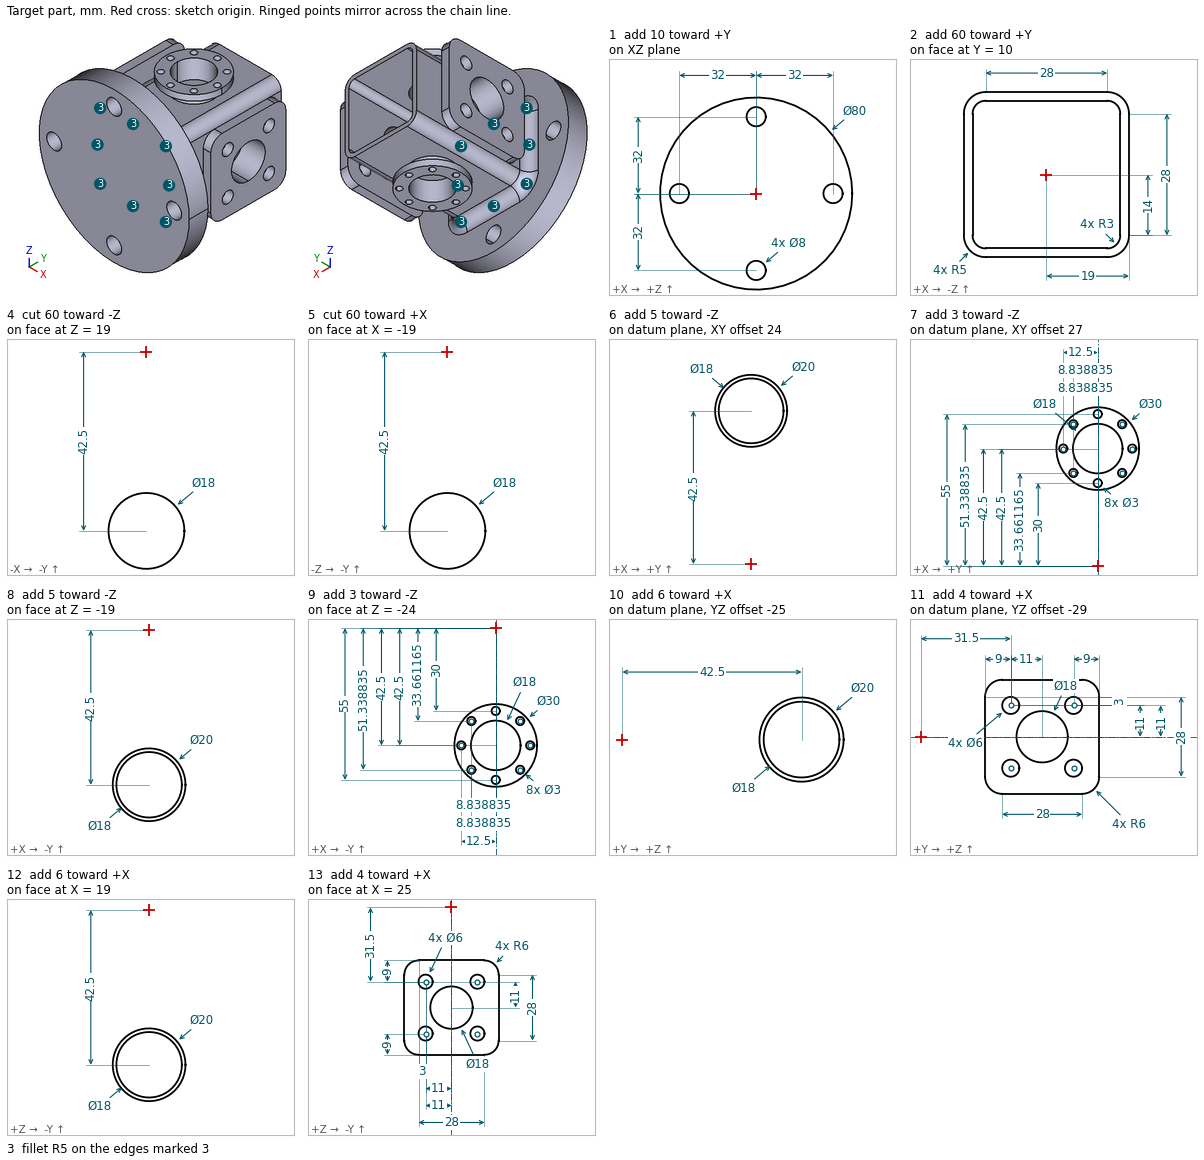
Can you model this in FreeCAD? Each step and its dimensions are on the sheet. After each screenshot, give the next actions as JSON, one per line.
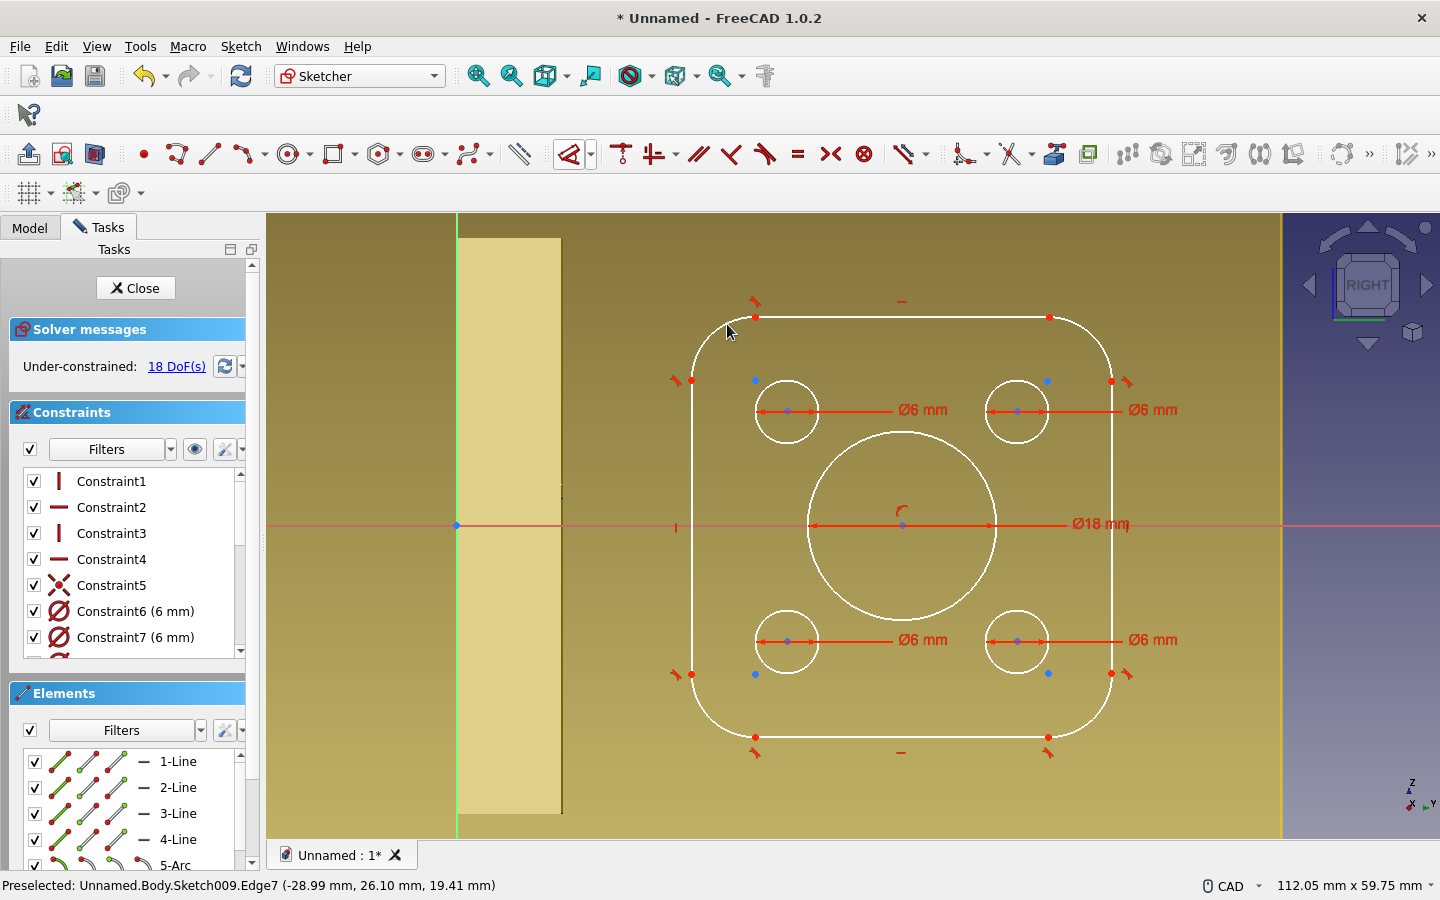
{"action": "left_click", "coordinate": [843, 317]}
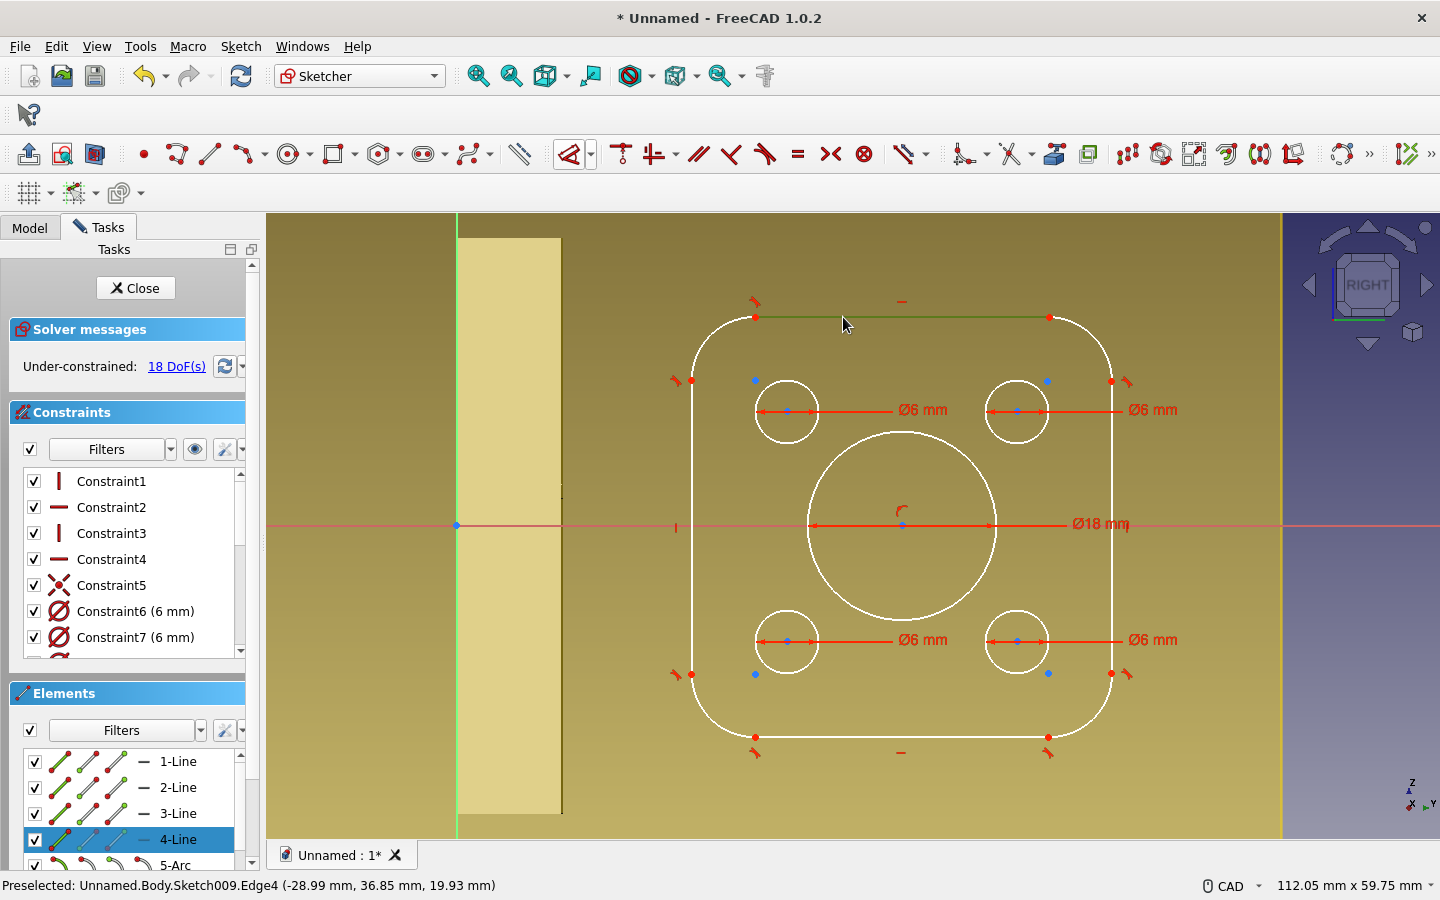
{"action": "left_click", "coordinate": [1105, 353]}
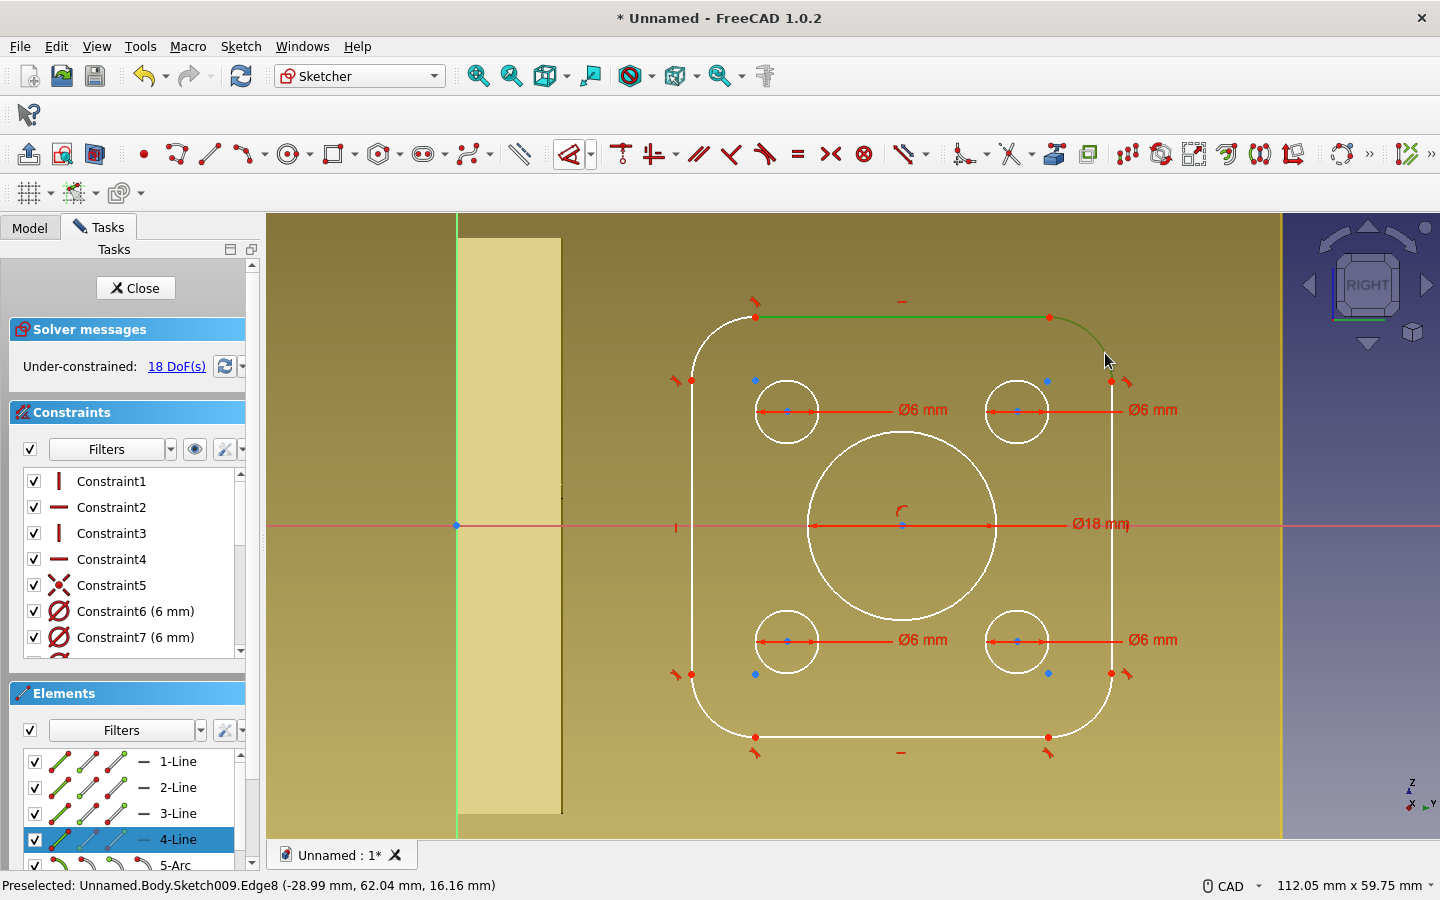
{"action": "key", "text": "t"}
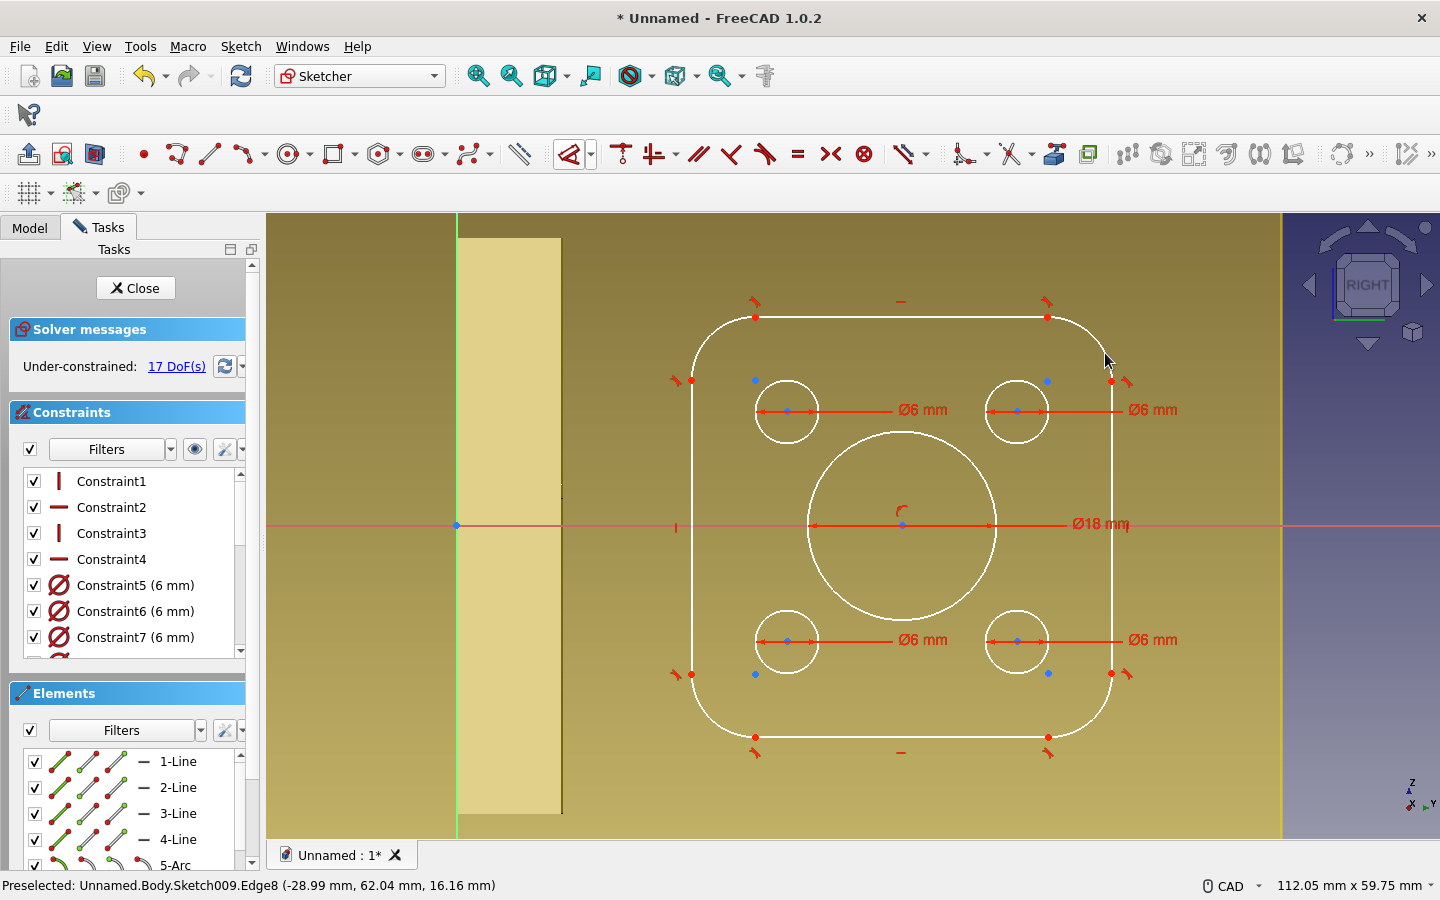
{"action": "left_click", "coordinate": [1077, 730]}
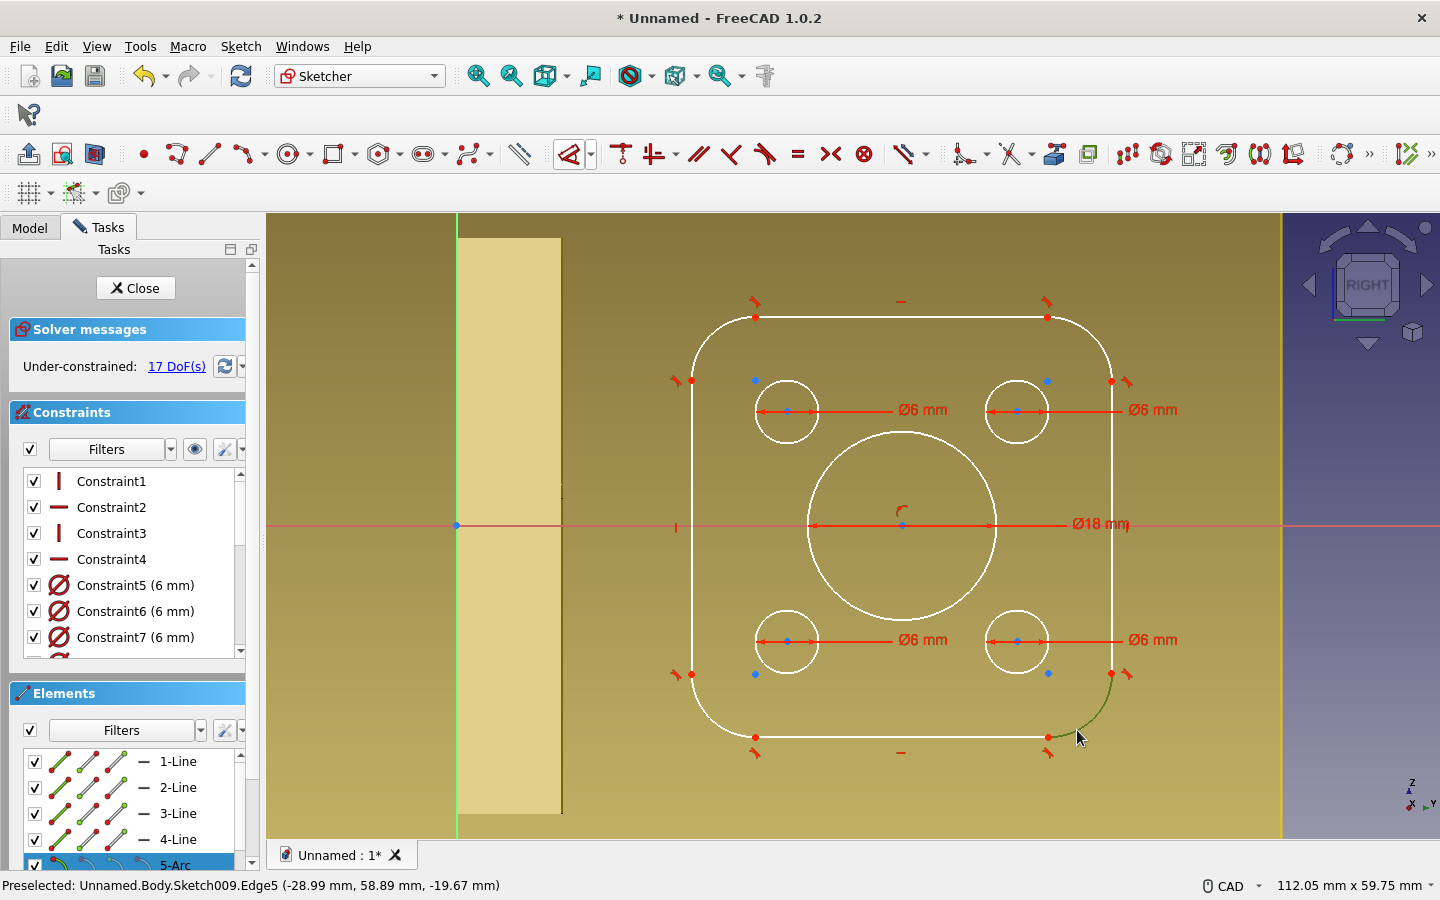
{"action": "left_click", "coordinate": [699, 703]}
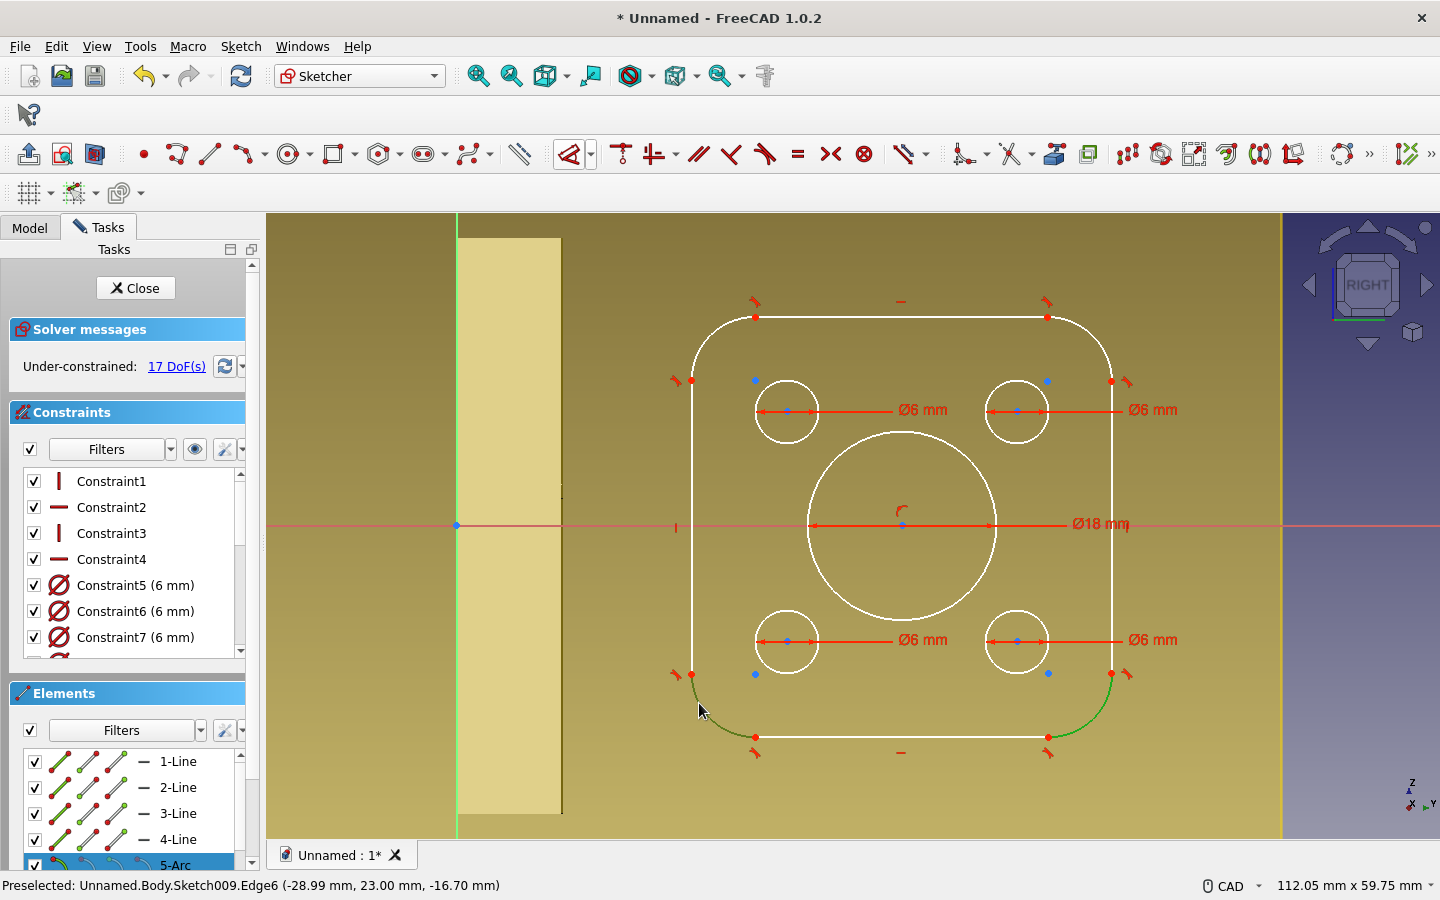
{"action": "left_click", "coordinate": [726, 324]}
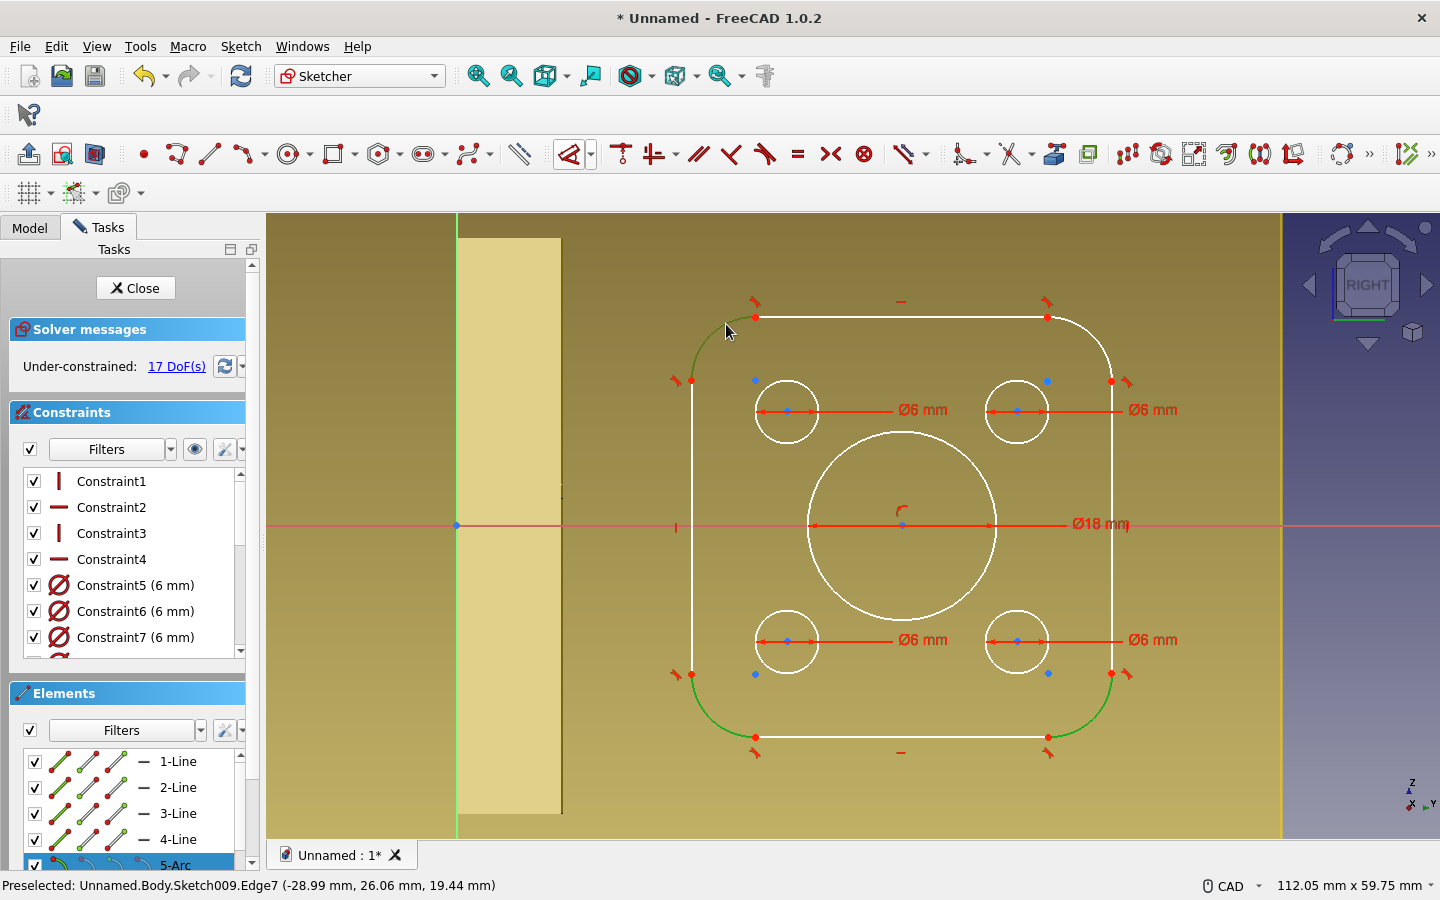
{"action": "left_click", "coordinate": [1105, 352]}